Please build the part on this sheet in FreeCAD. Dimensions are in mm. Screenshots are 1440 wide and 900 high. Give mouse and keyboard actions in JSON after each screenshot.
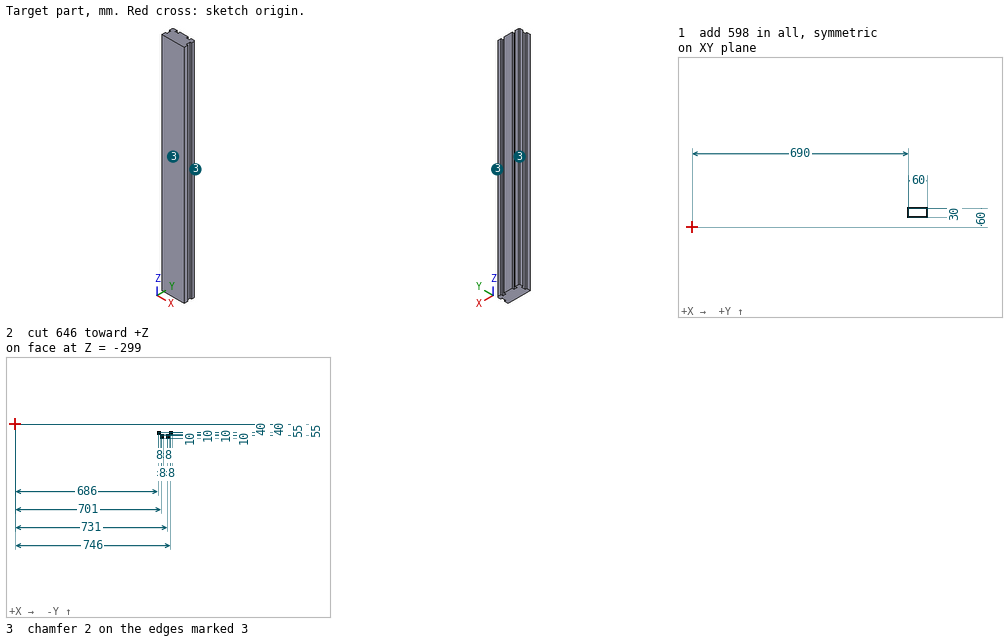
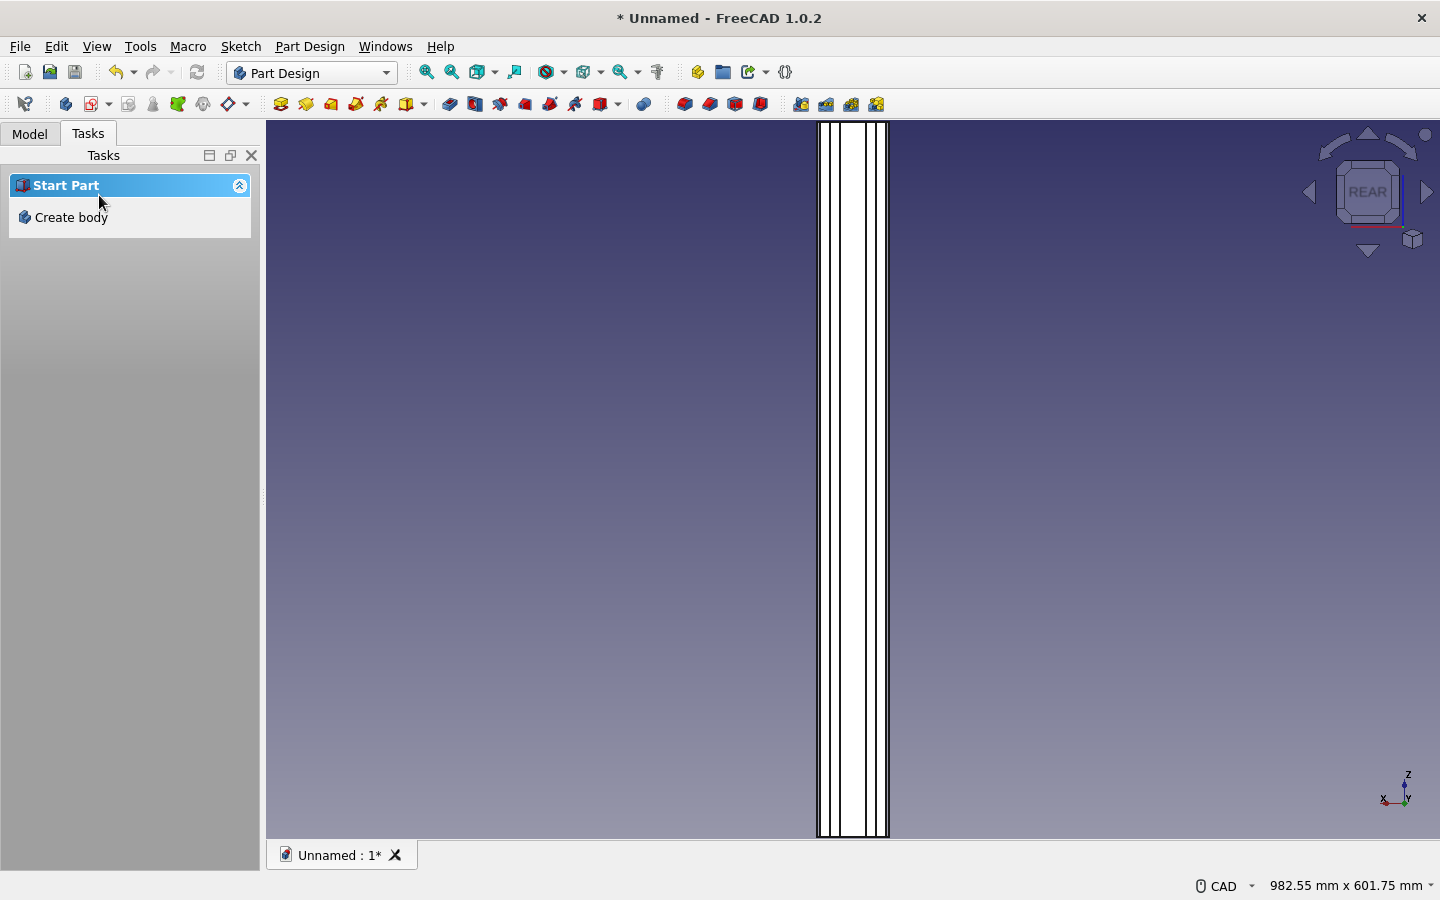
{"action": "key", "text": "0"}